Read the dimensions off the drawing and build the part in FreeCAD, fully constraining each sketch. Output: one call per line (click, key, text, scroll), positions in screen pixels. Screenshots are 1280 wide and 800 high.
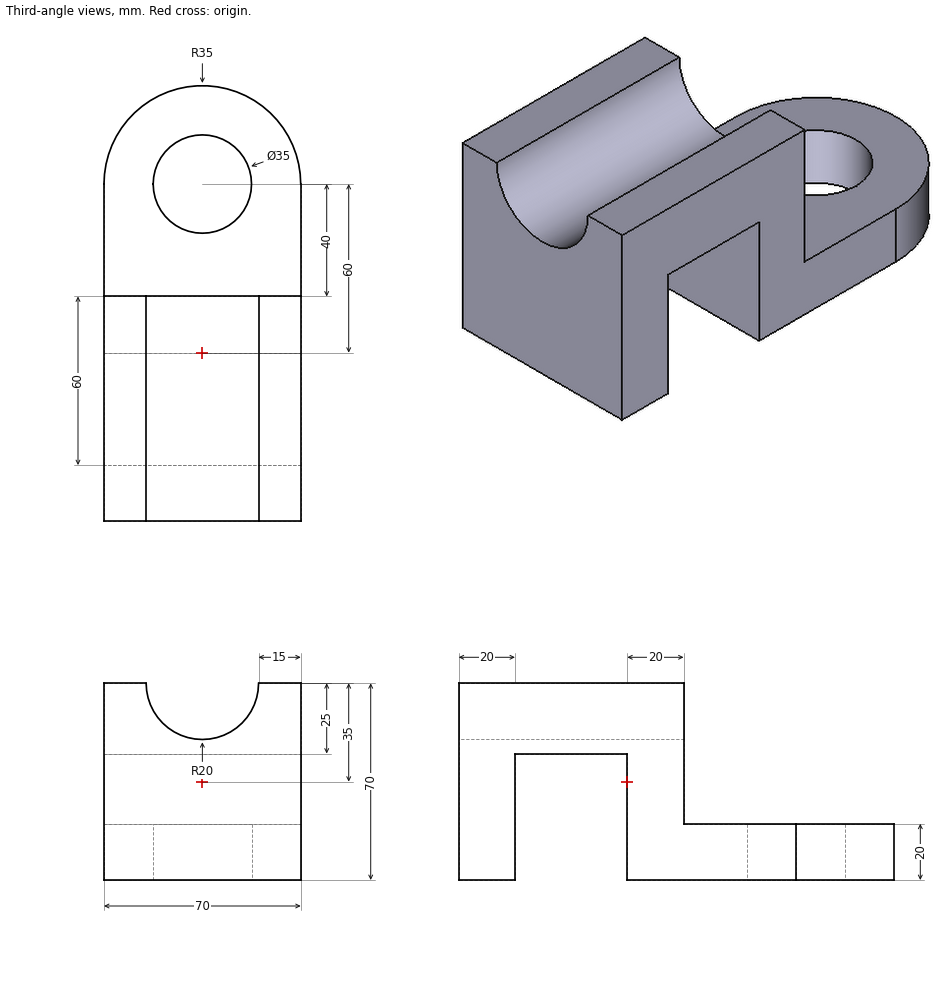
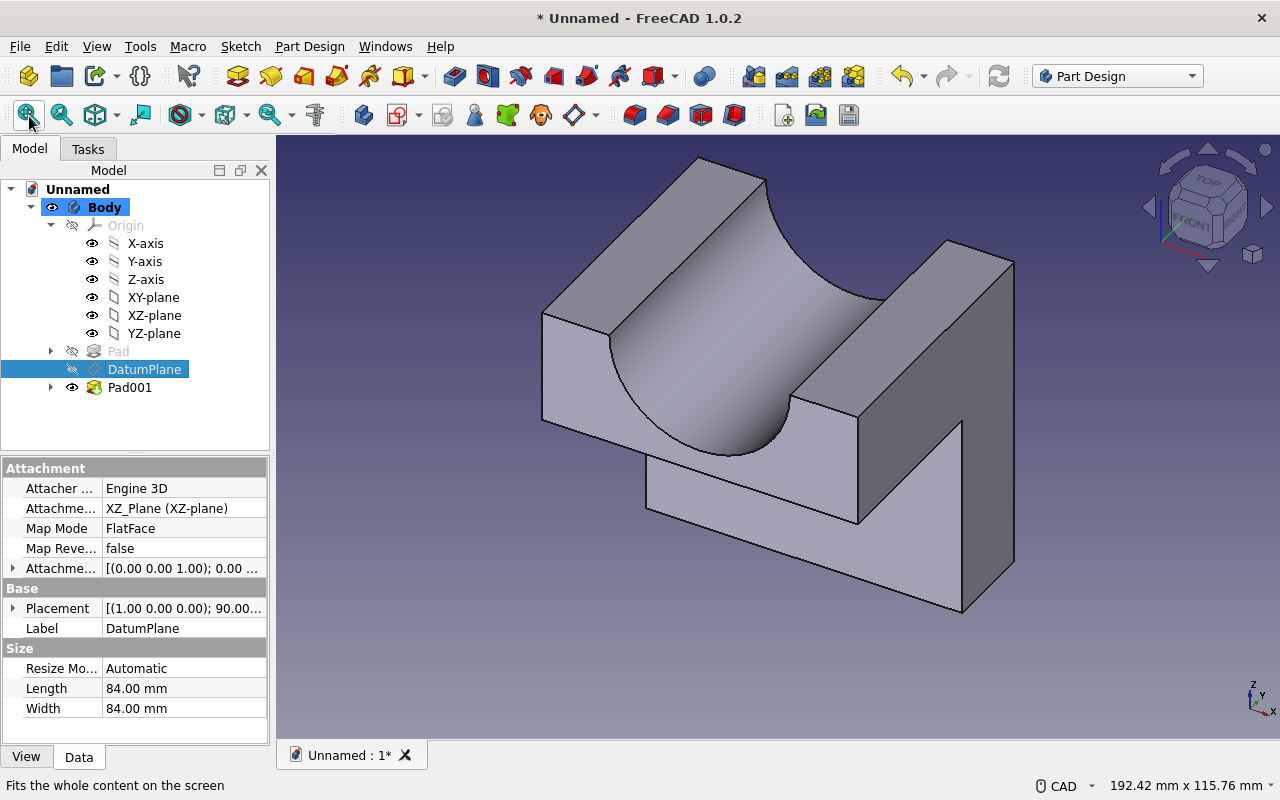
click(137, 315)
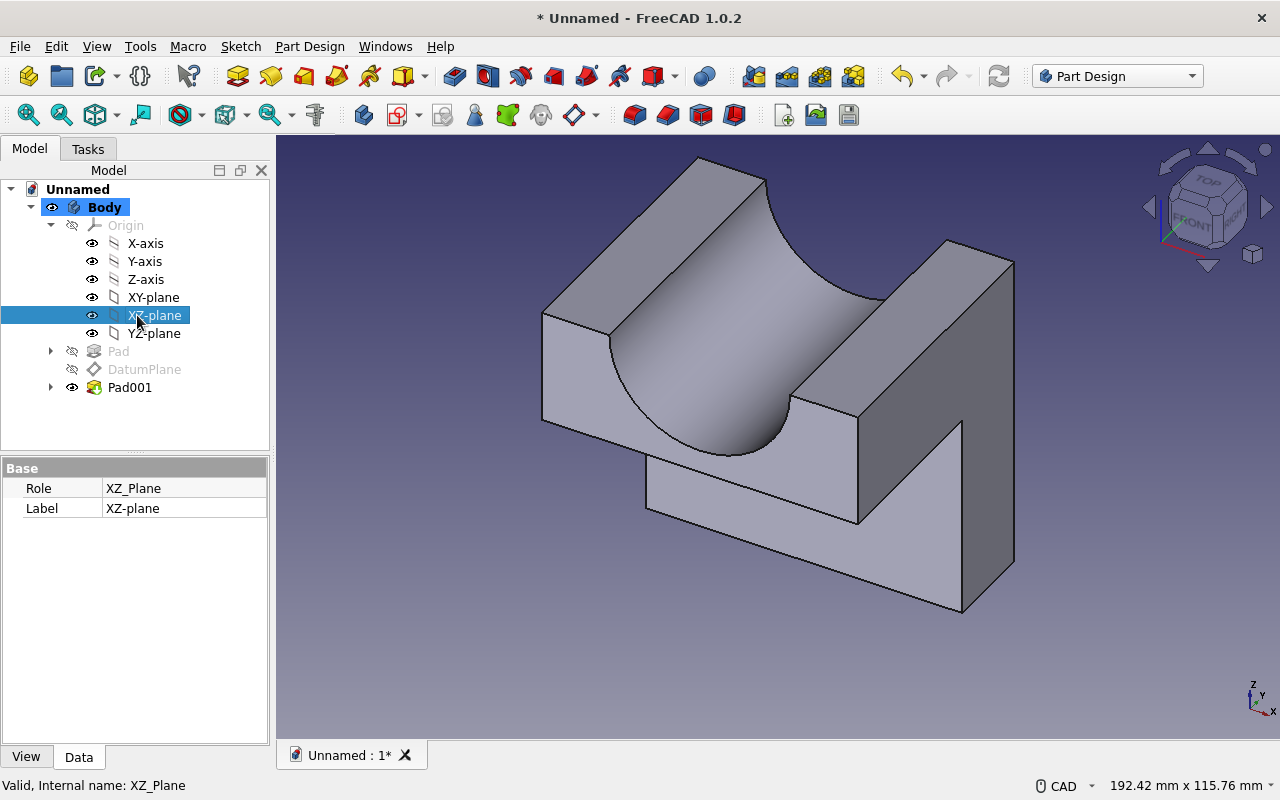
click(574, 116)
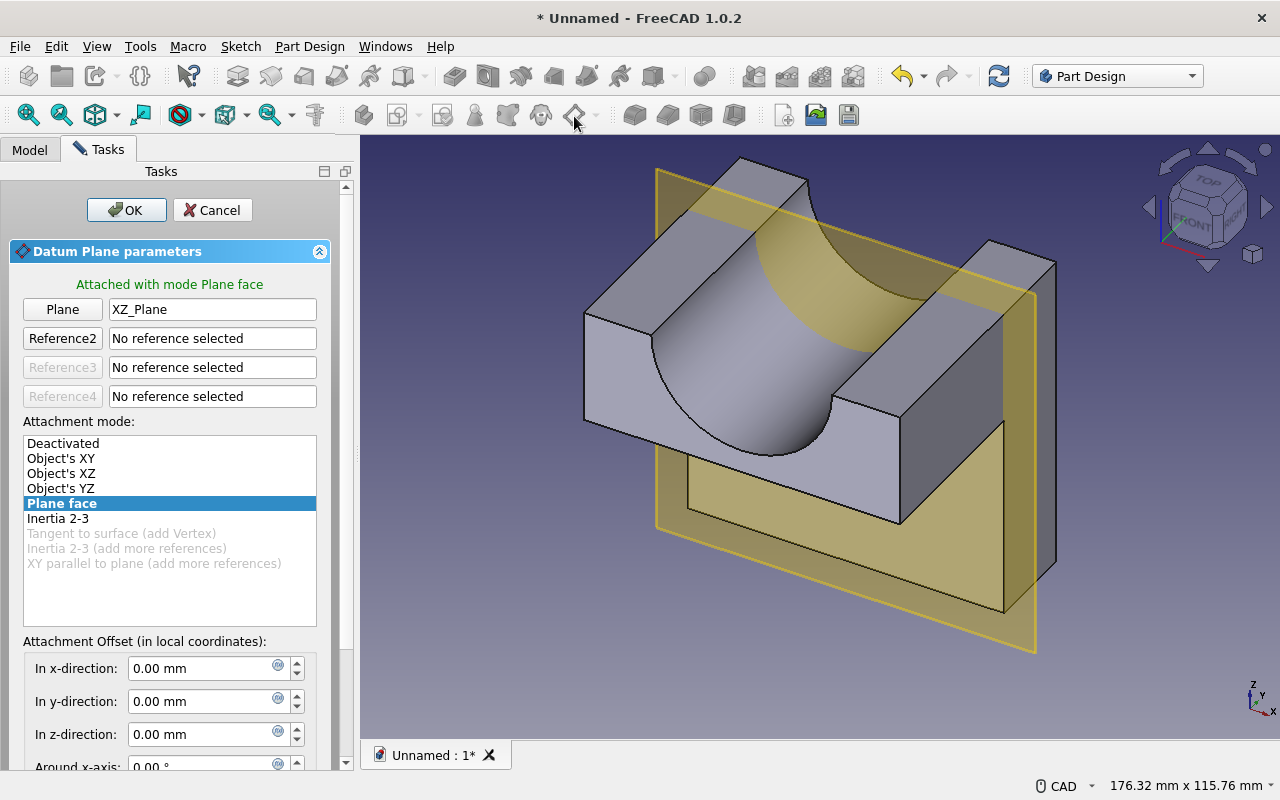
triple_click(210, 734)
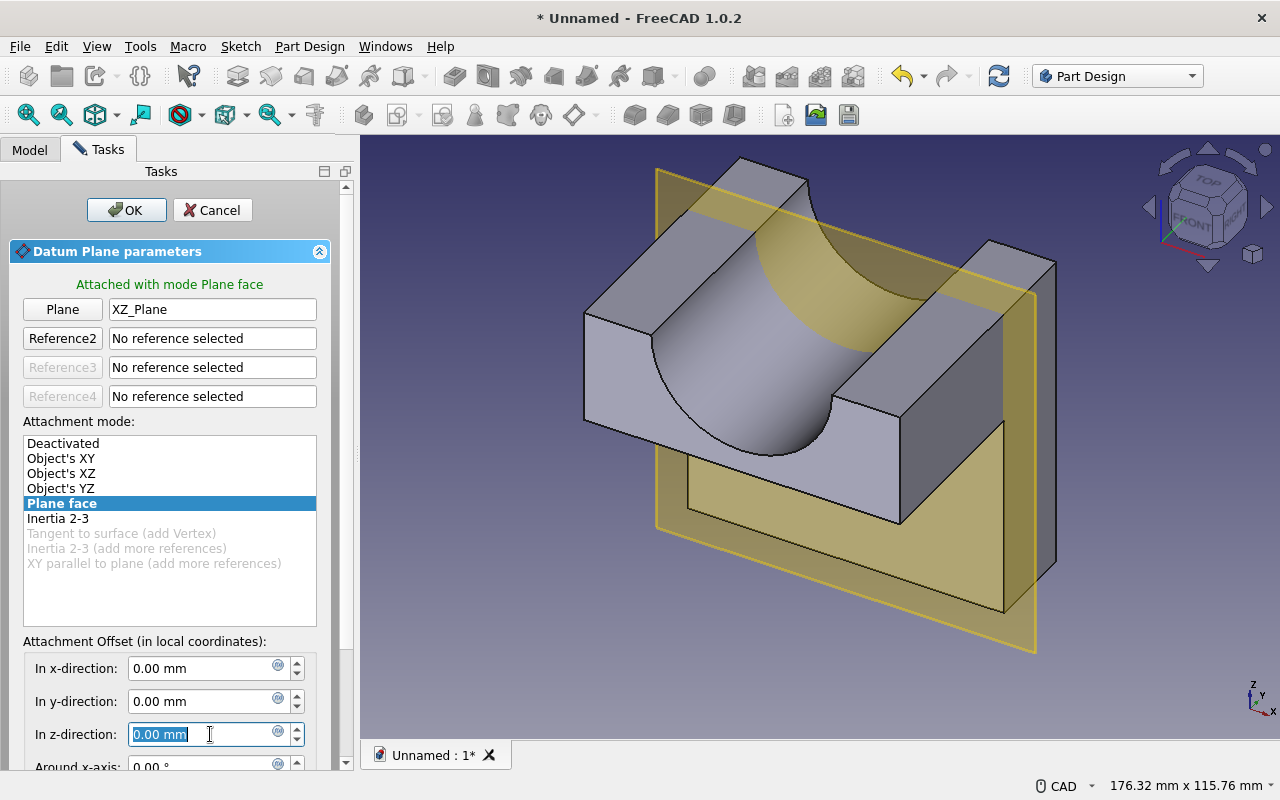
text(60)
key(Tab)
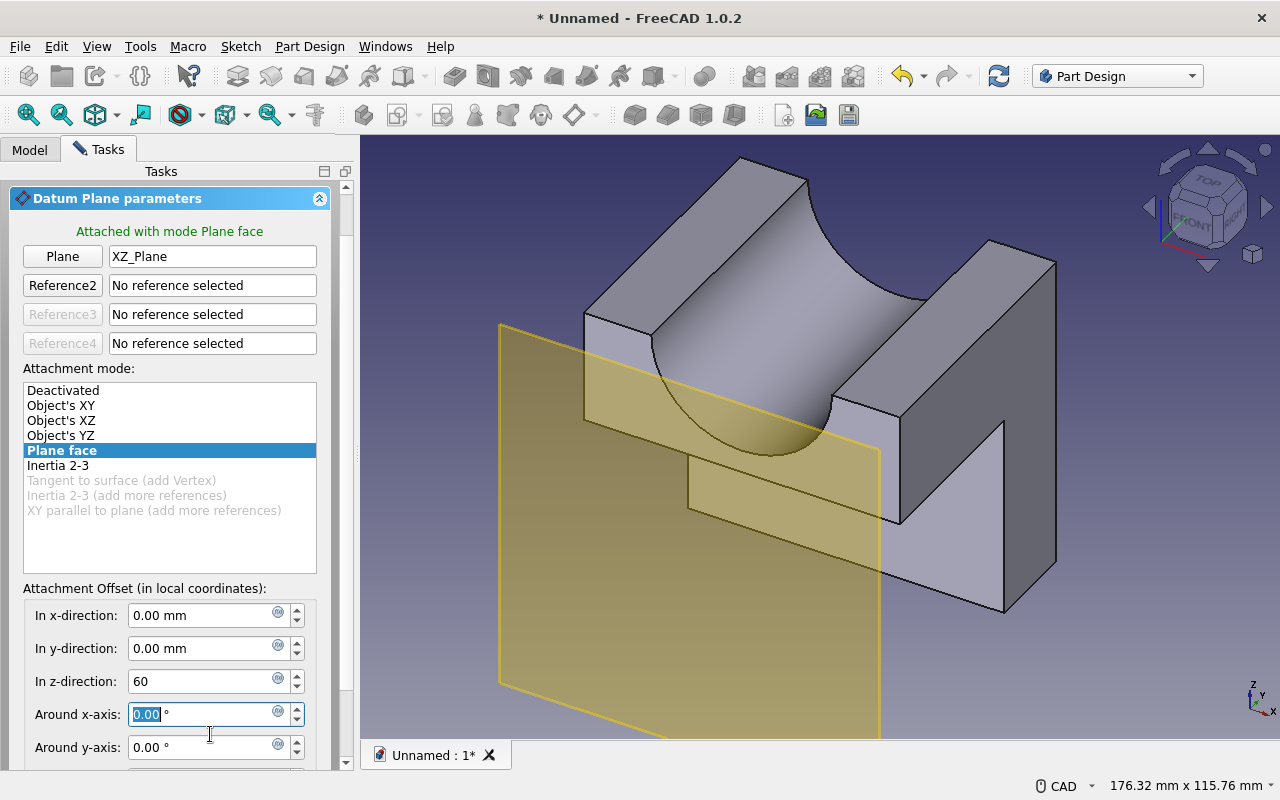
scroll(346, 476, up, 2)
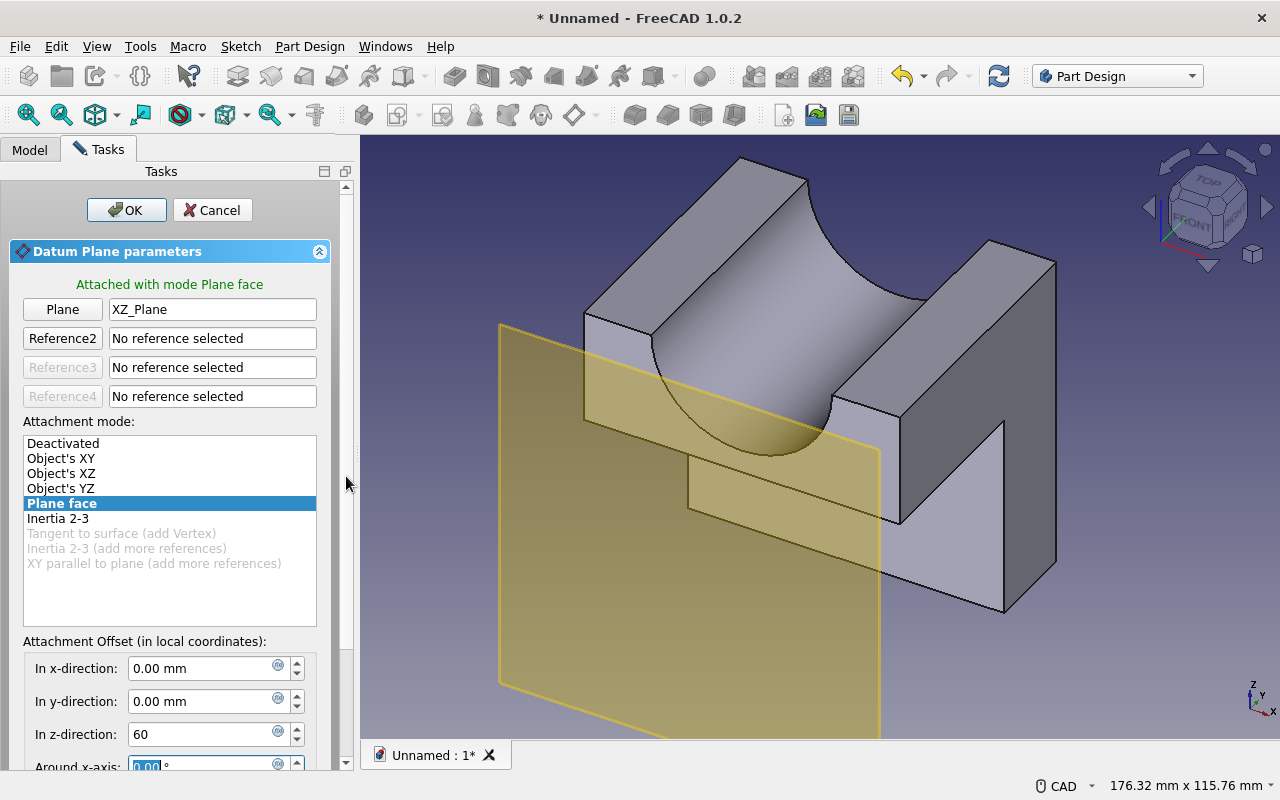
click(127, 210)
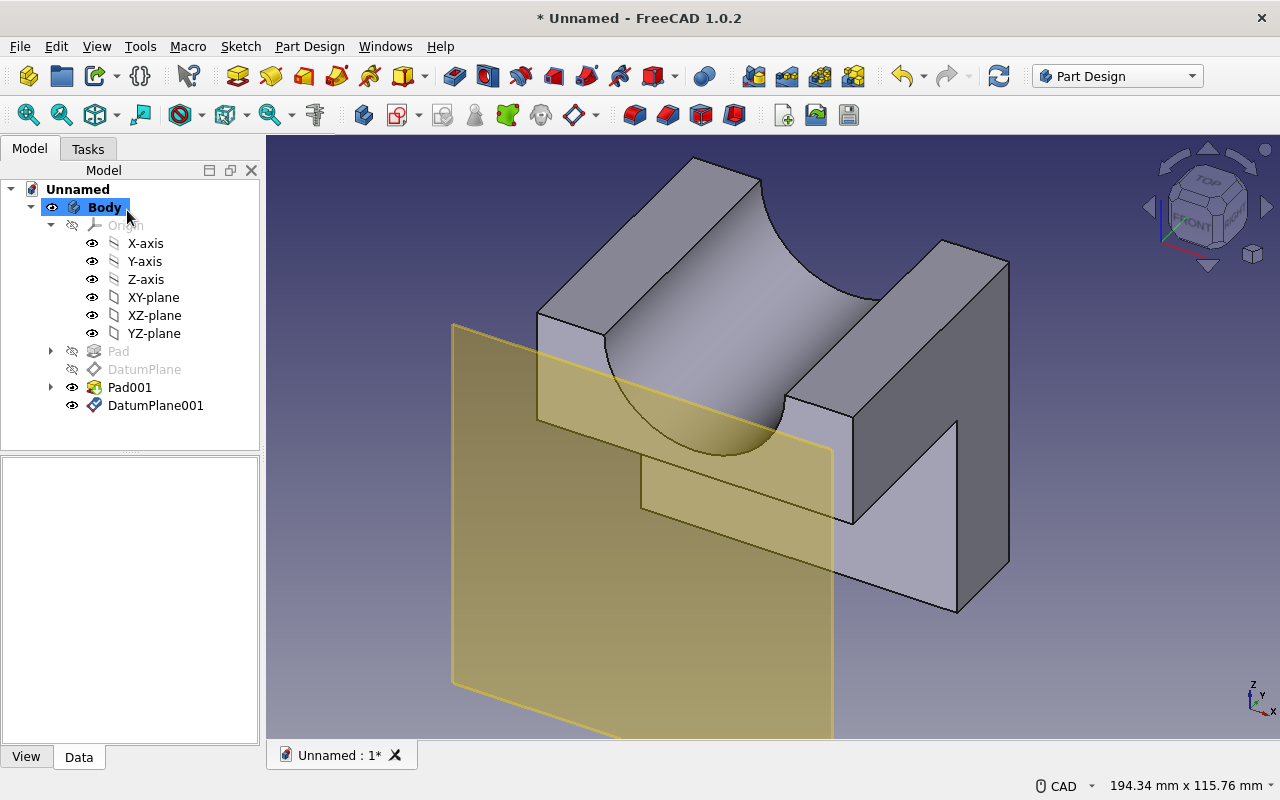
click(117, 405)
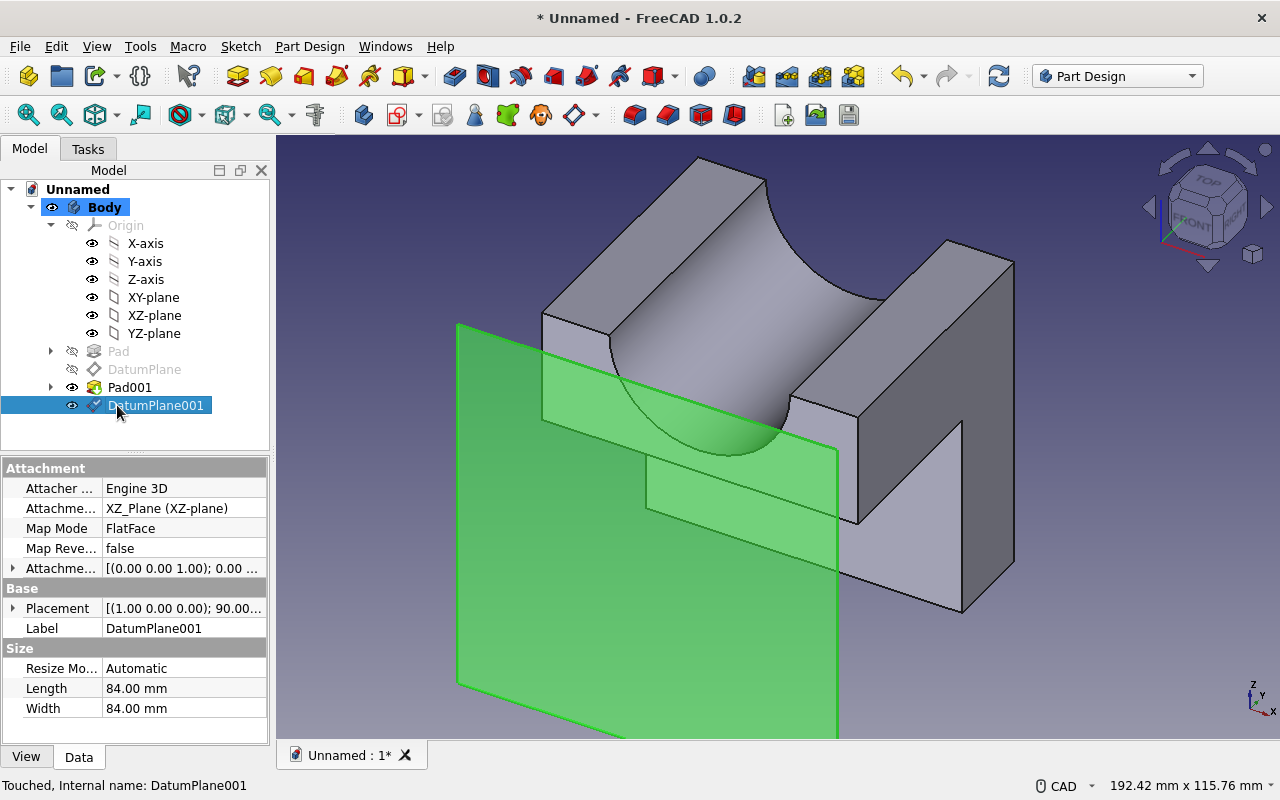
click(396, 116)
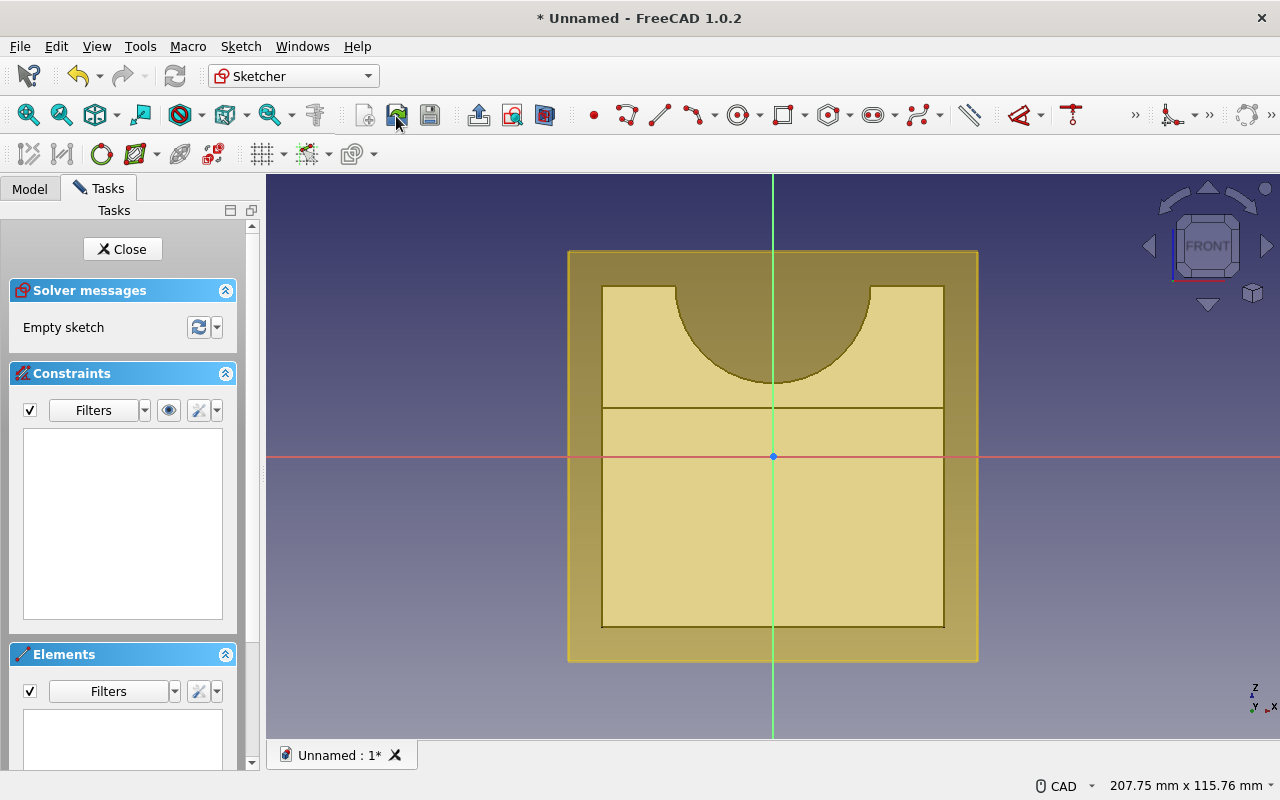
click(627, 116)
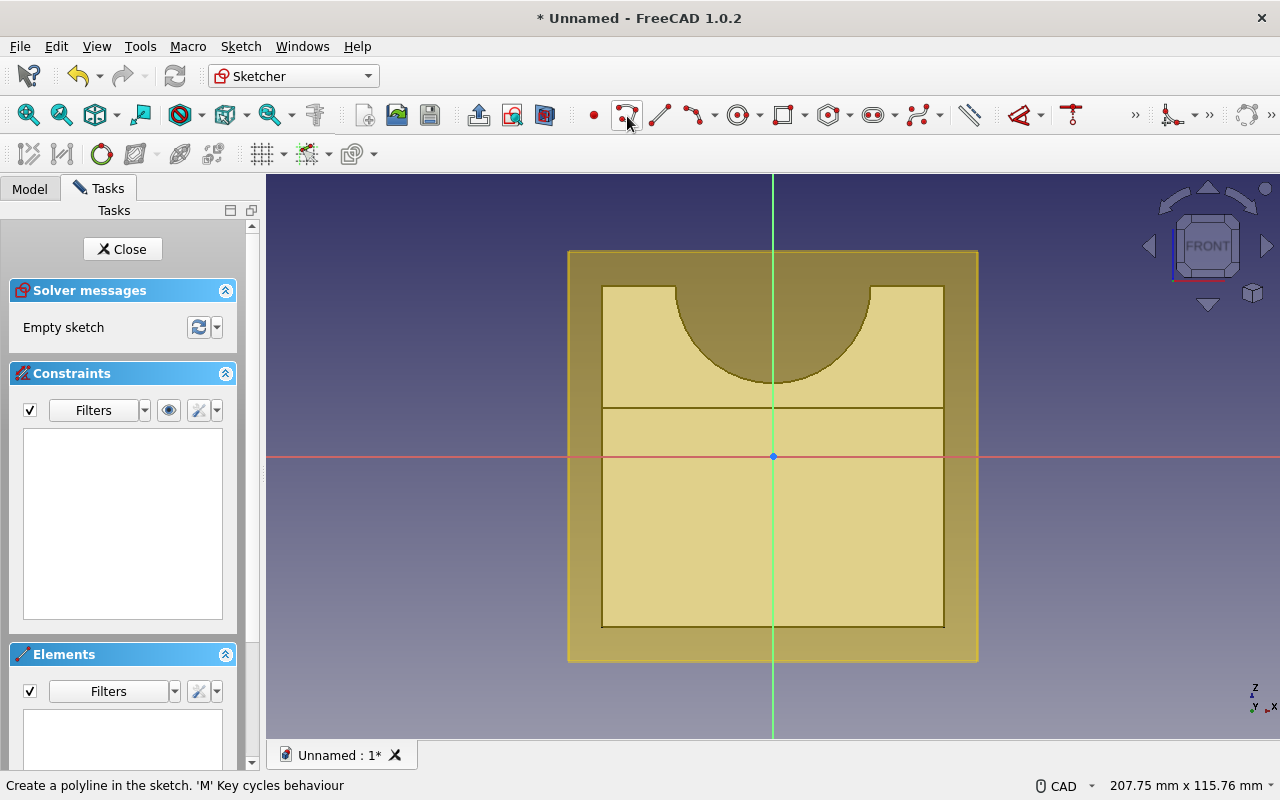
click(871, 286)
click(944, 286)
click(944, 627)
click(602, 627)
click(602, 286)
click(675, 286)
right_click(675, 286)